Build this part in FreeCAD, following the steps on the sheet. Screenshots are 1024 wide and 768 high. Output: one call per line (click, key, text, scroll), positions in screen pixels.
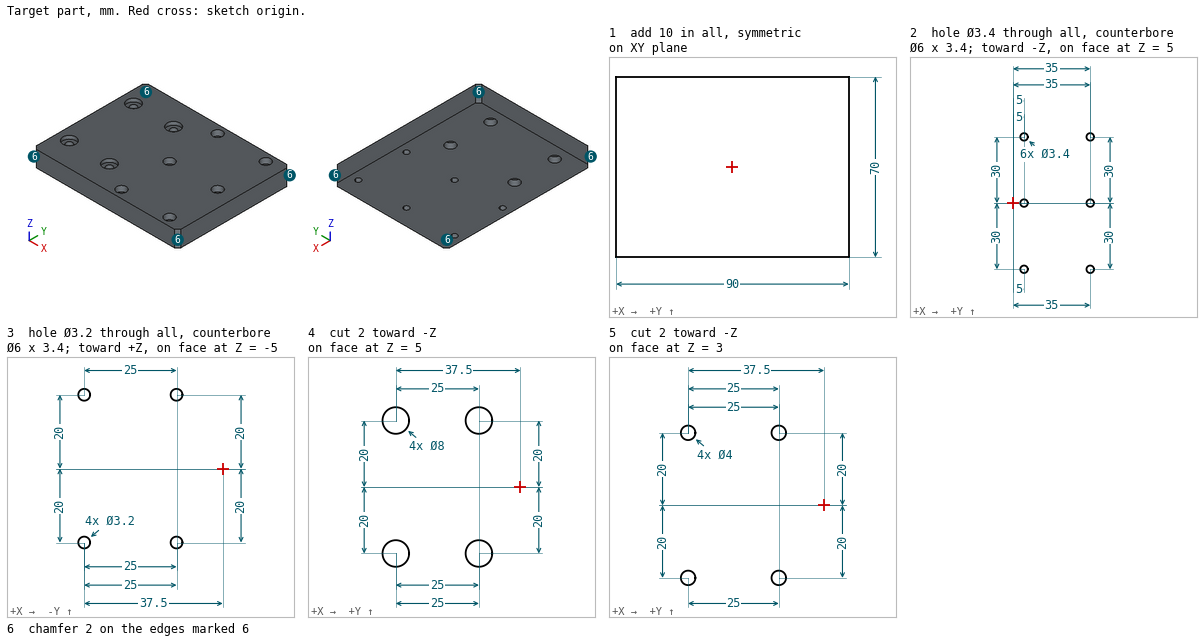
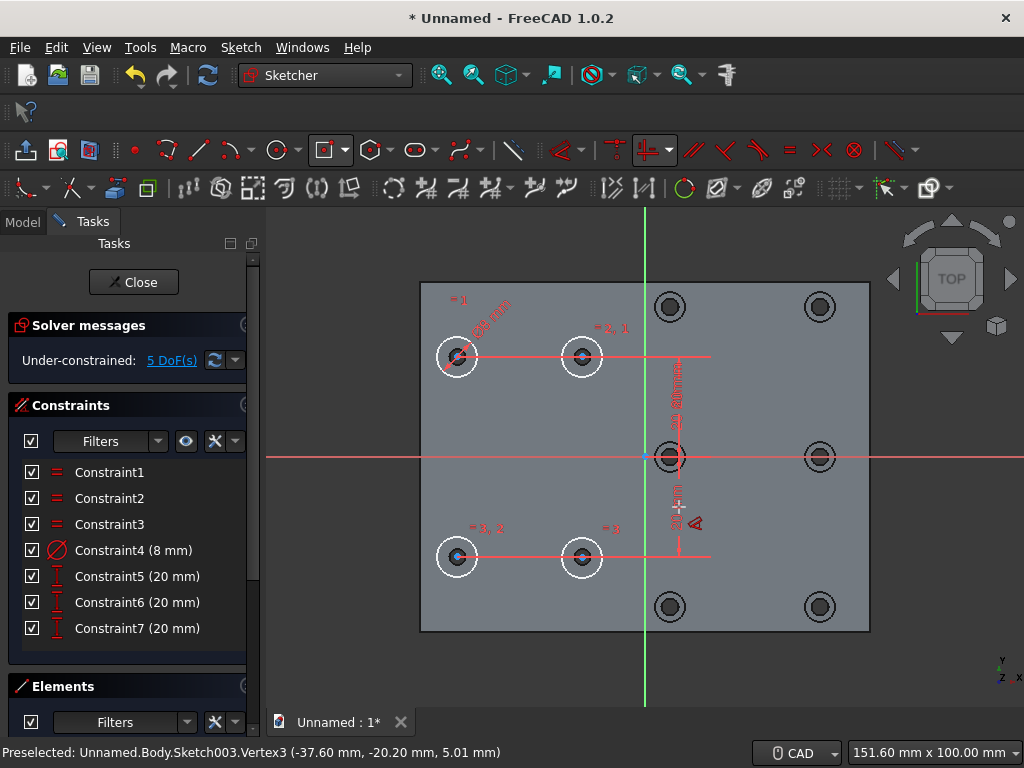
click(582, 558)
click(679, 484)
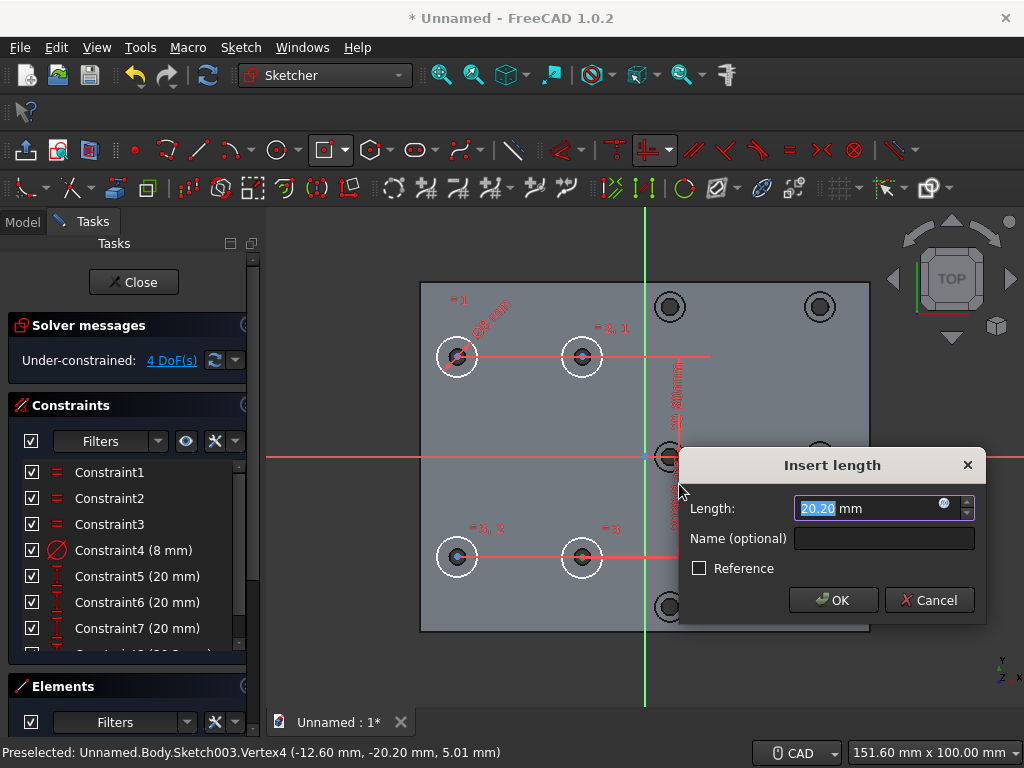
text(20)
key(Return)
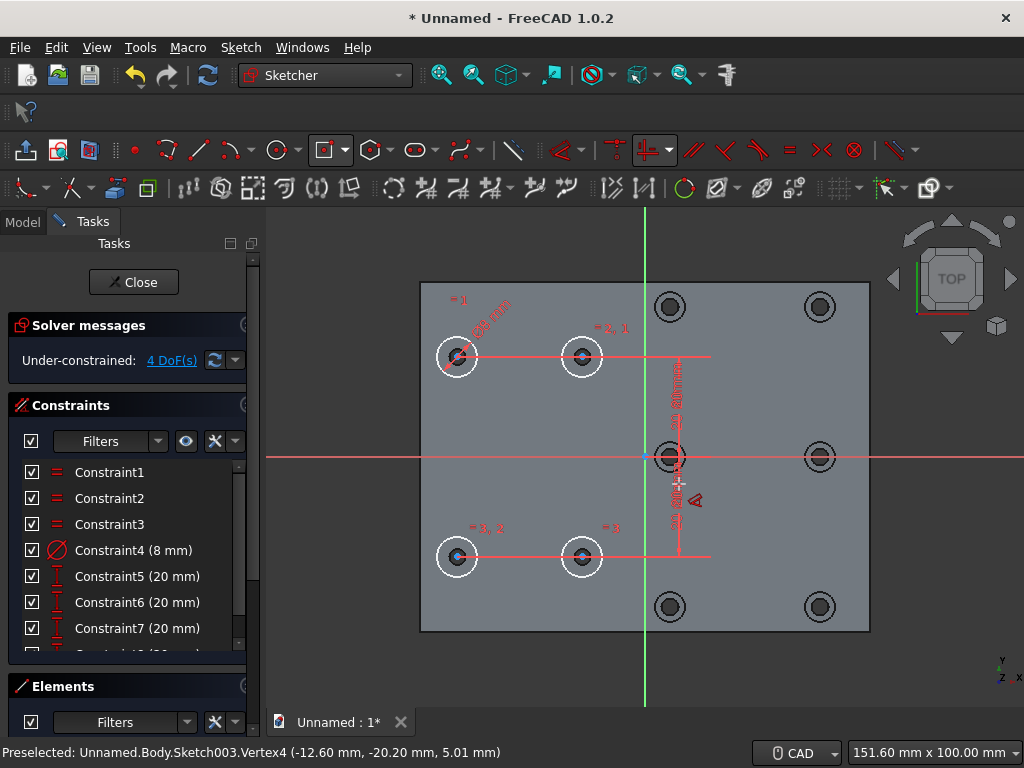
click(457, 357)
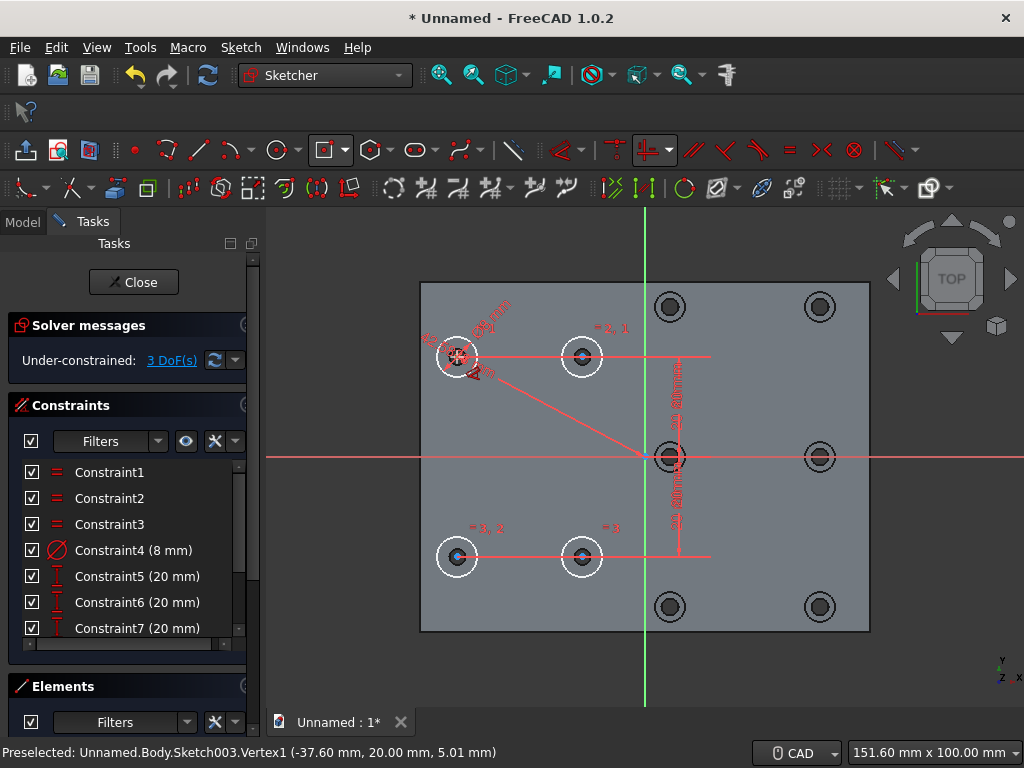
click(582, 357)
click(563, 323)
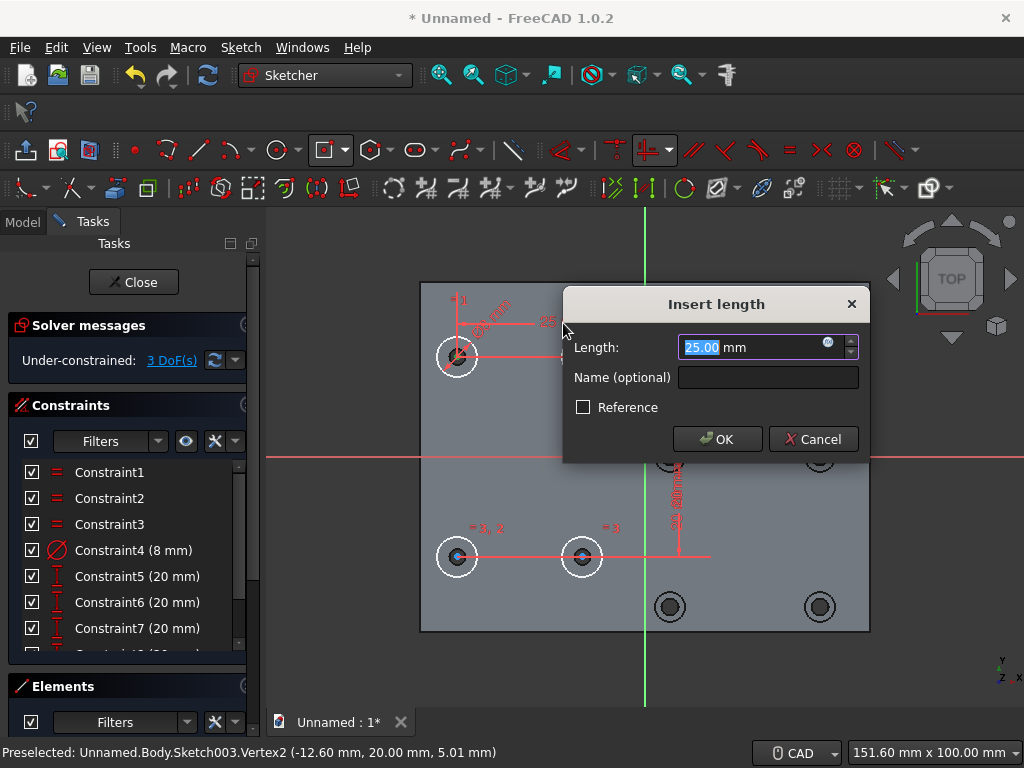
text(25)
key(Return)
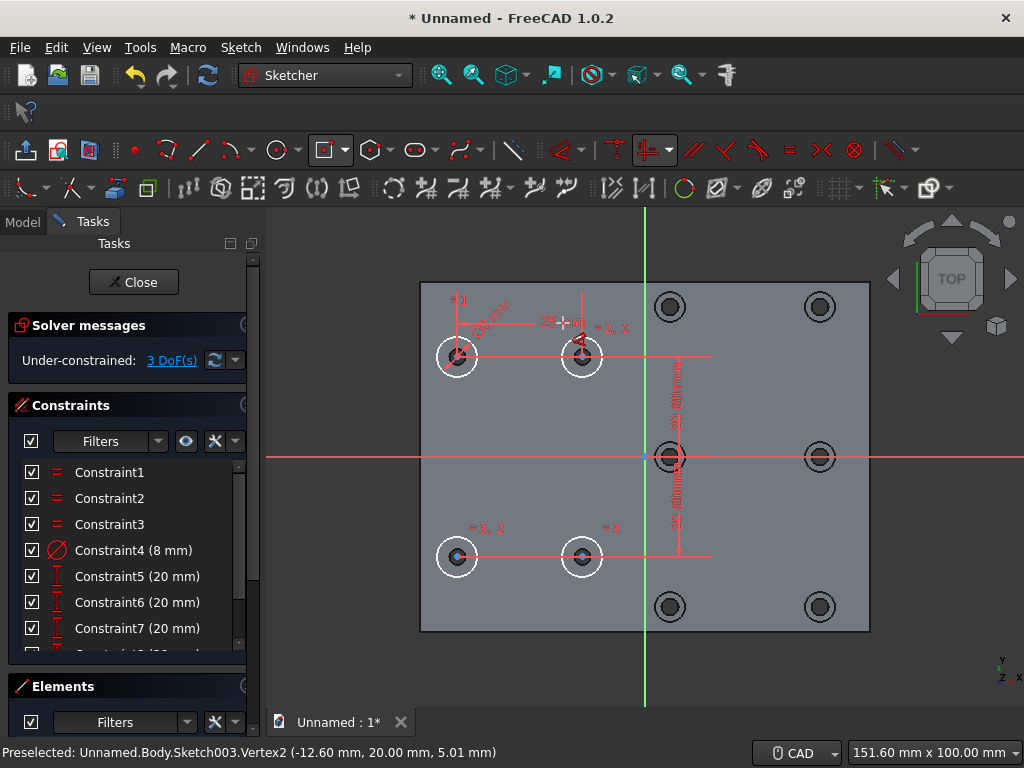
click(582, 357)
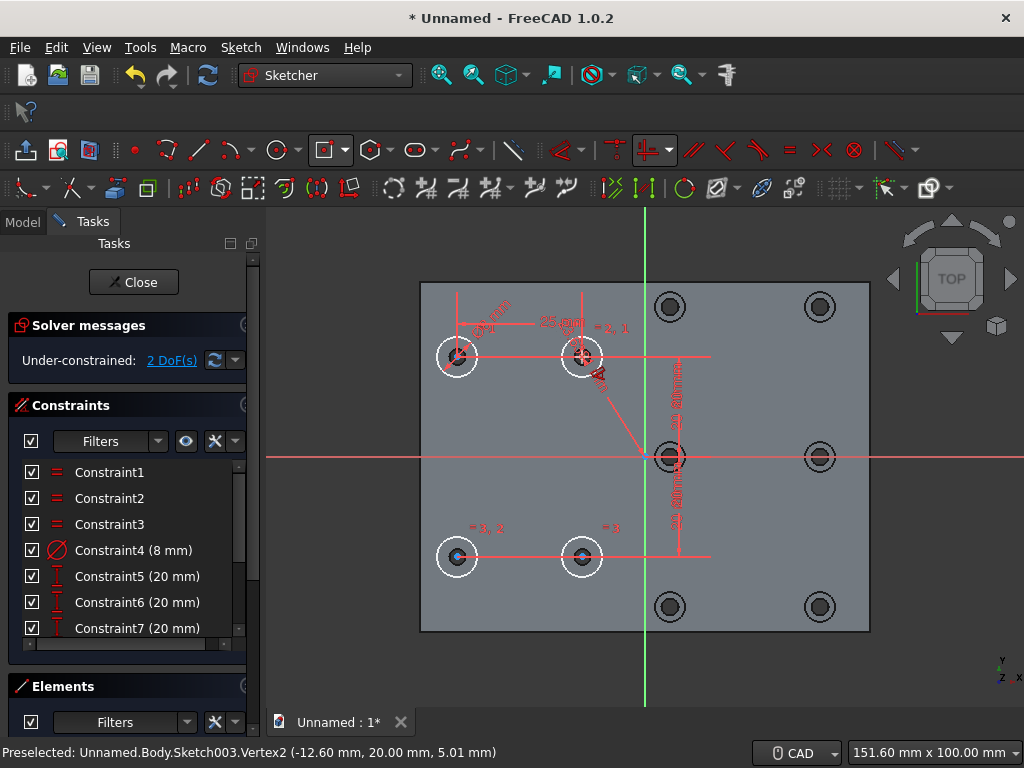
click(457, 557)
click(519, 591)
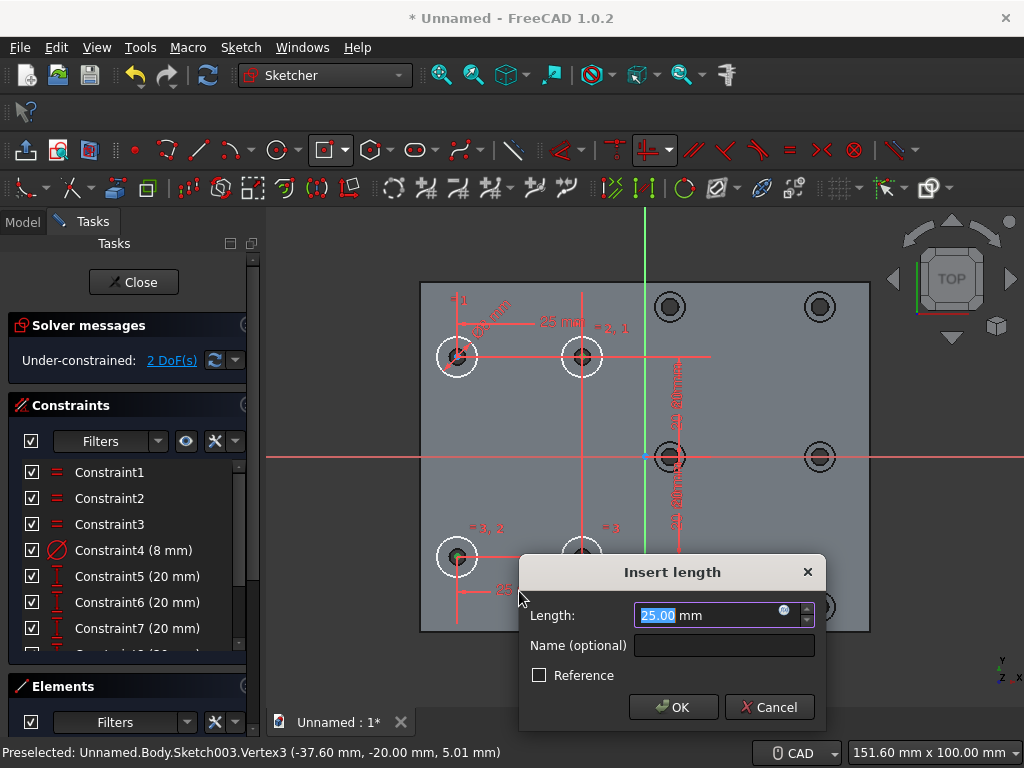
text(25)
key(Return)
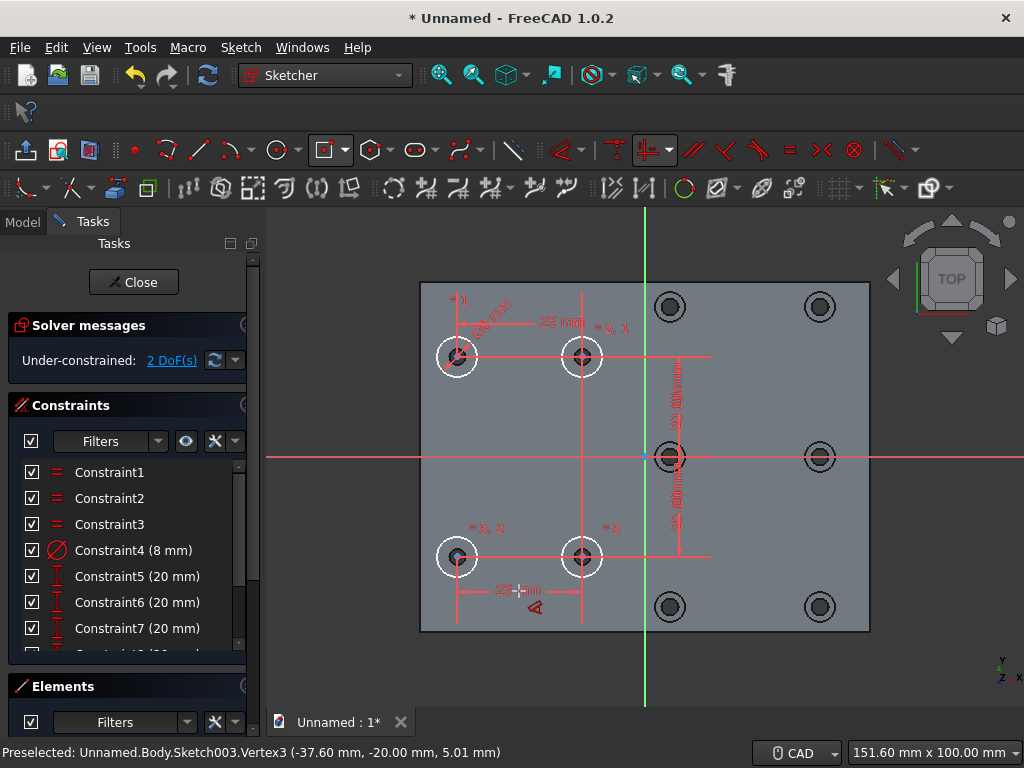
click(457, 557)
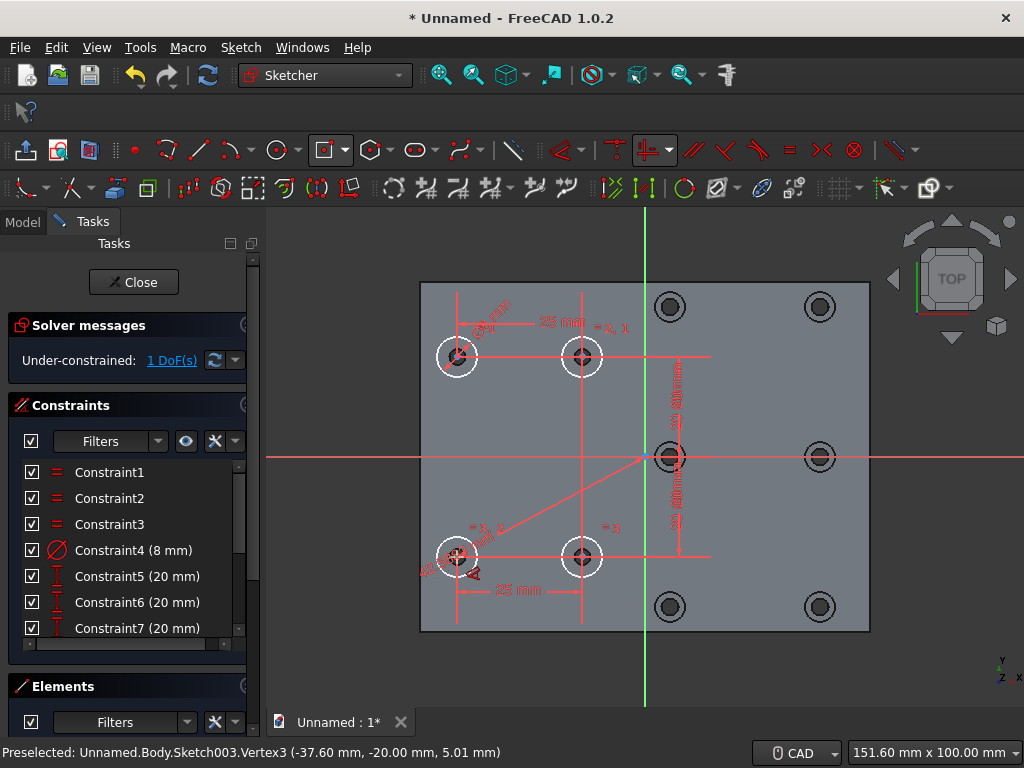
click(582, 557)
click(519, 523)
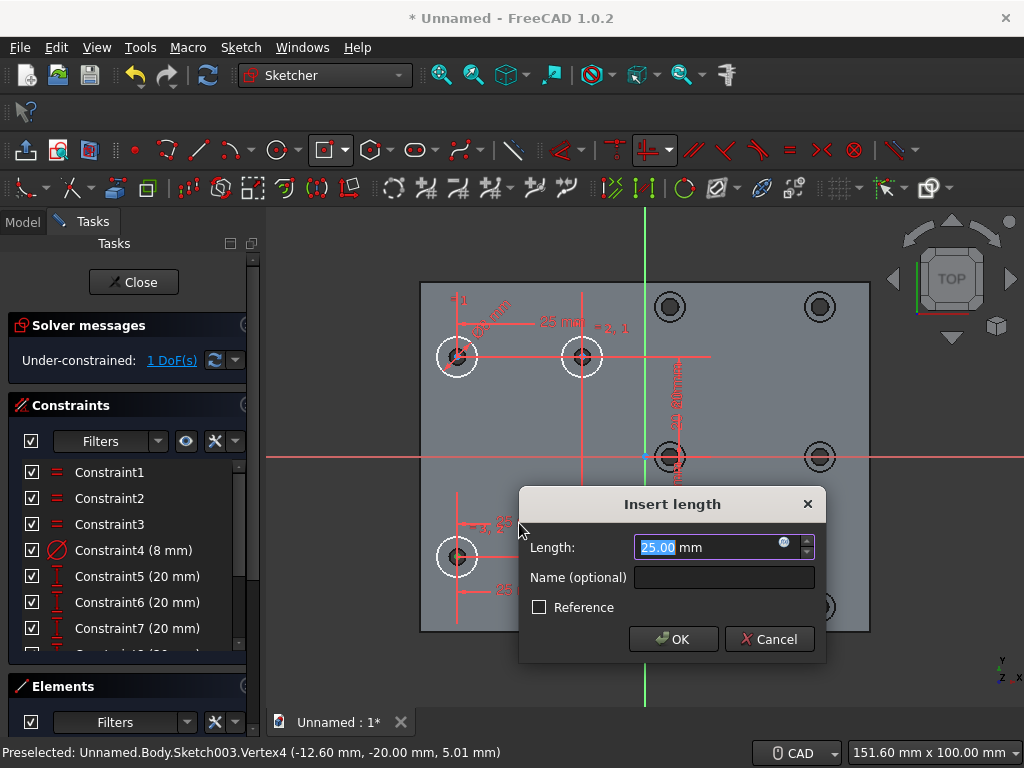
text(25)
key(Return)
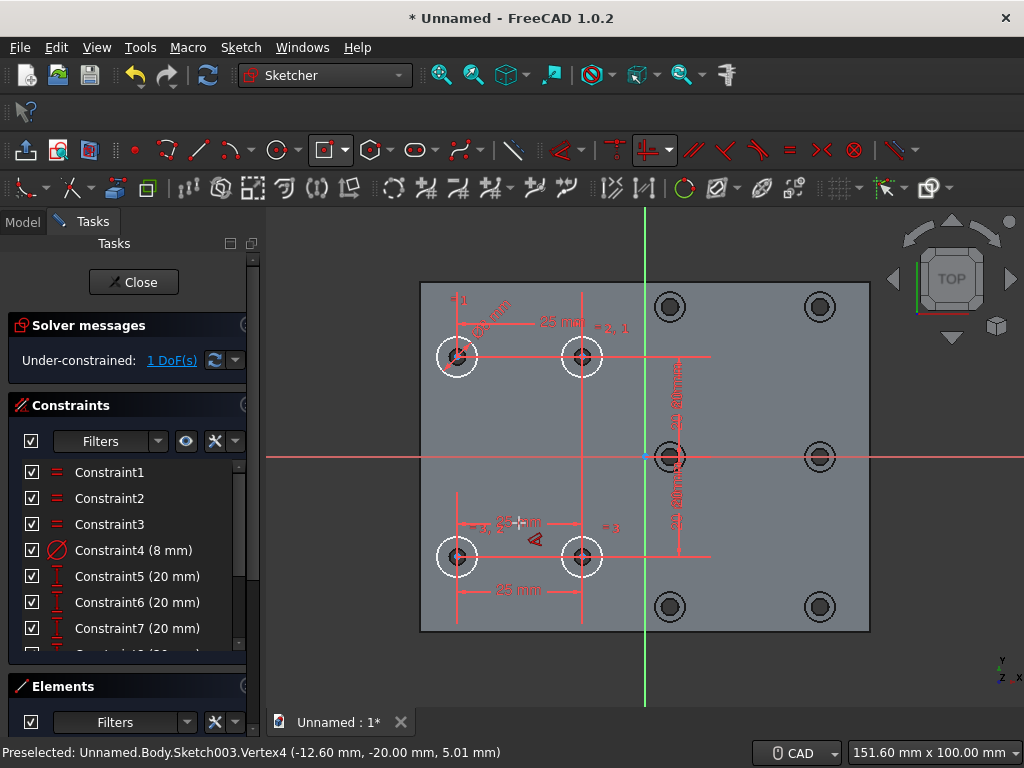
click(457, 357)
click(551, 491)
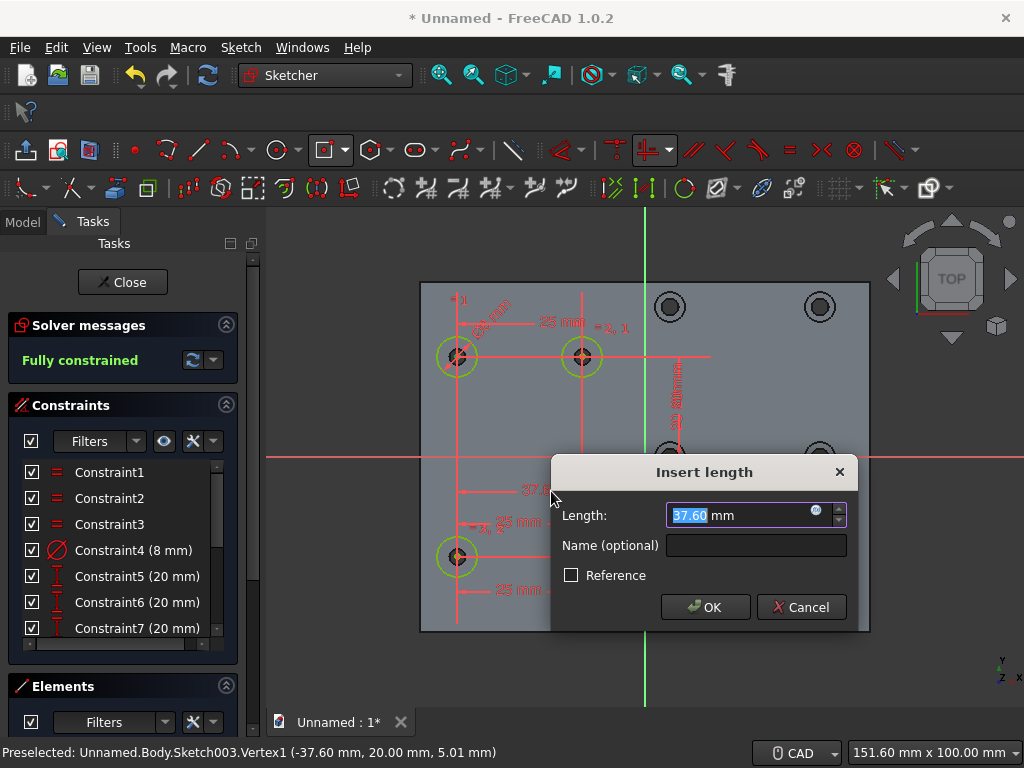
text(37.5)
key(Return)
key(Escape)